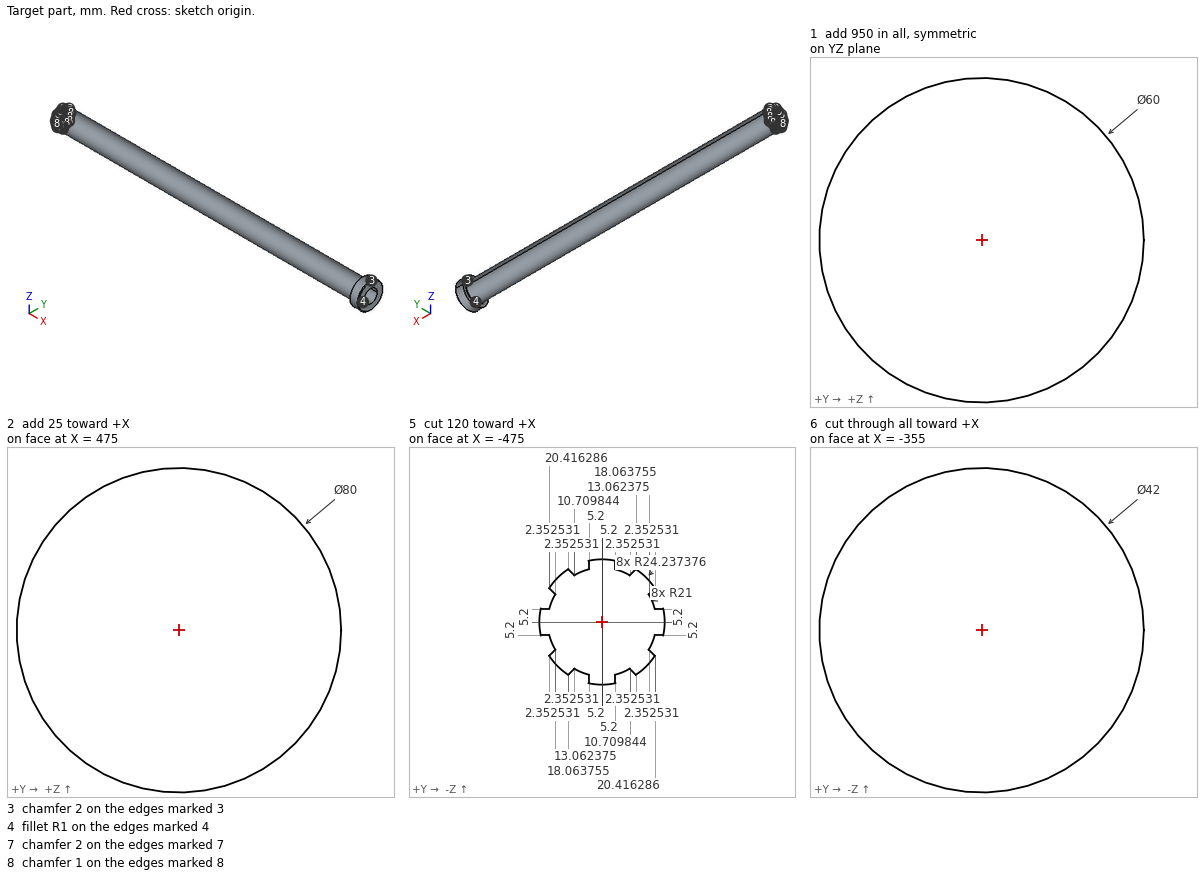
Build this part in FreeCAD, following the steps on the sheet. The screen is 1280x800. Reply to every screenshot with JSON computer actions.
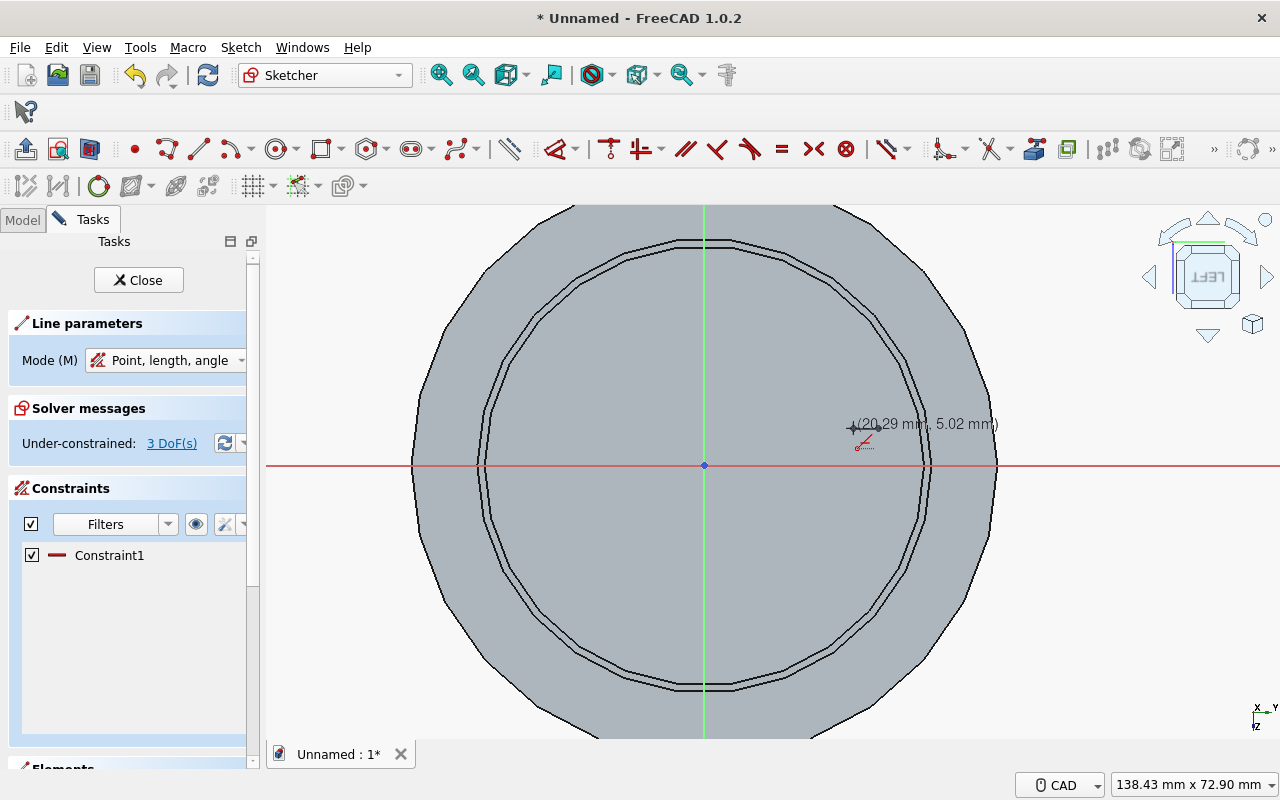
{"action": "left_click", "coordinate": [837, 387]}
{"action": "left_click", "coordinate": [854, 370]}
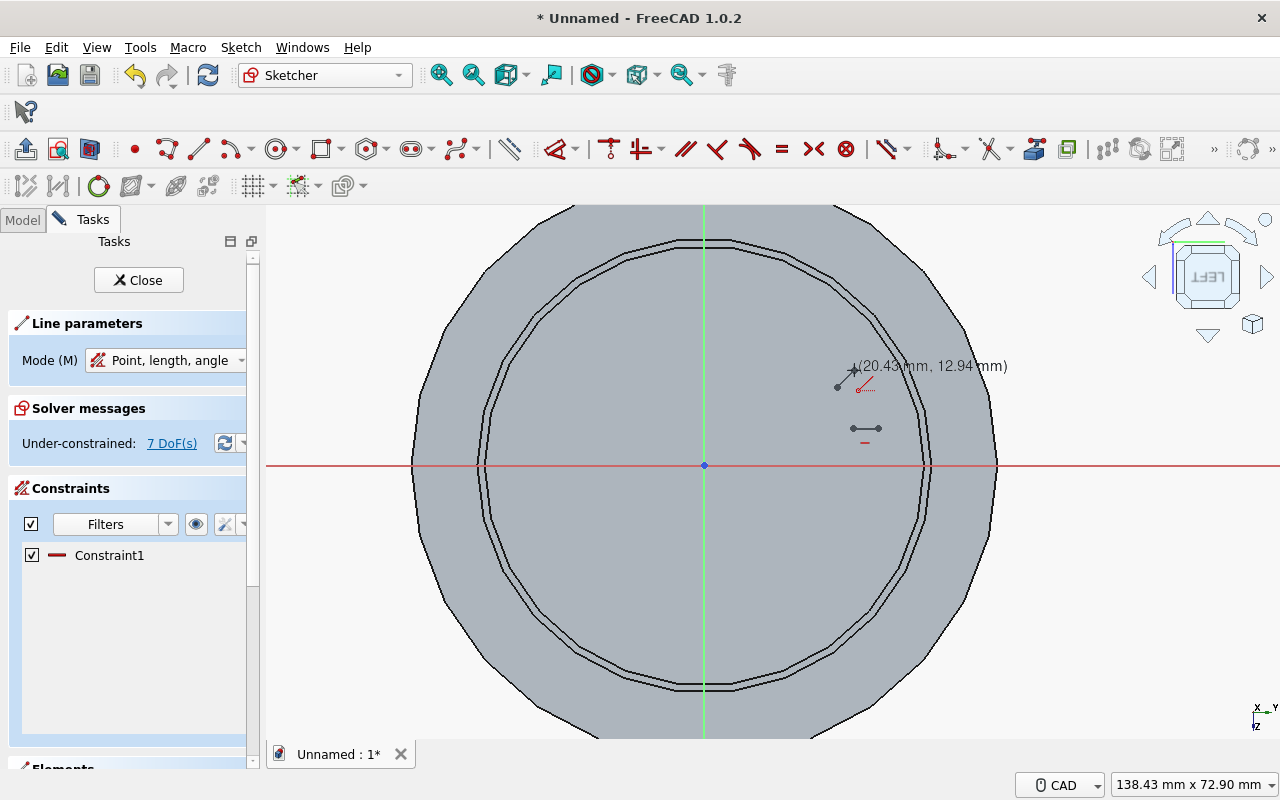
{"action": "left_click", "coordinate": [800, 316]}
{"action": "left_click", "coordinate": [783, 333]}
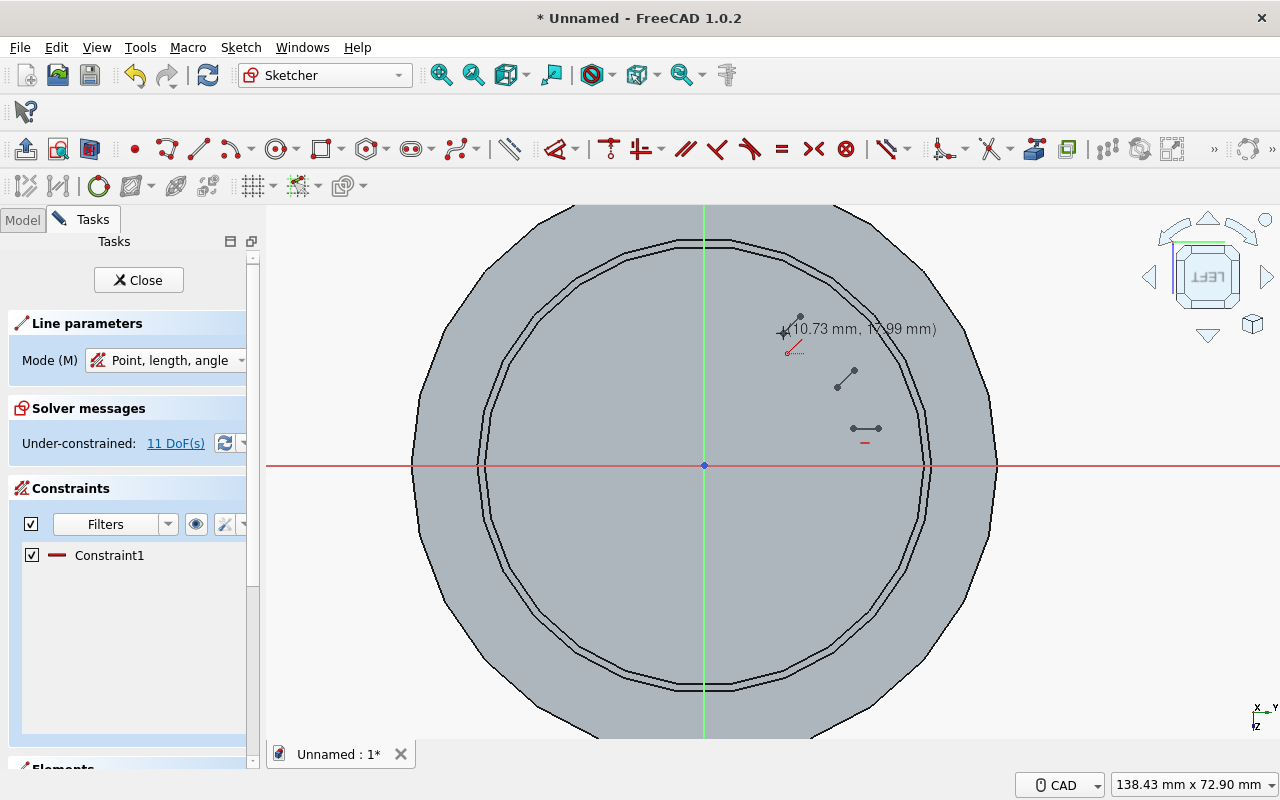
{"action": "left_click", "coordinate": [742, 317]}
{"action": "left_click", "coordinate": [742, 292]}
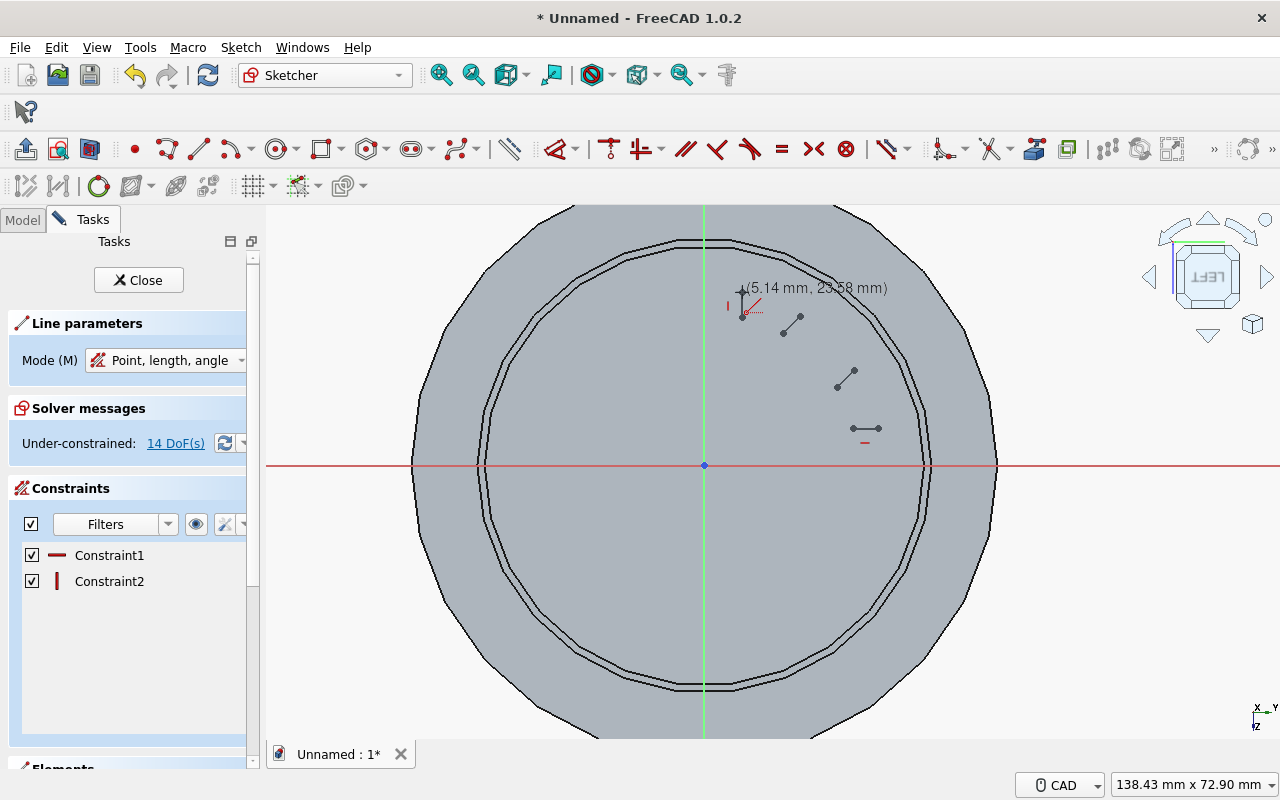
{"action": "left_click", "coordinate": [666, 292]}
{"action": "left_click", "coordinate": [666, 317]}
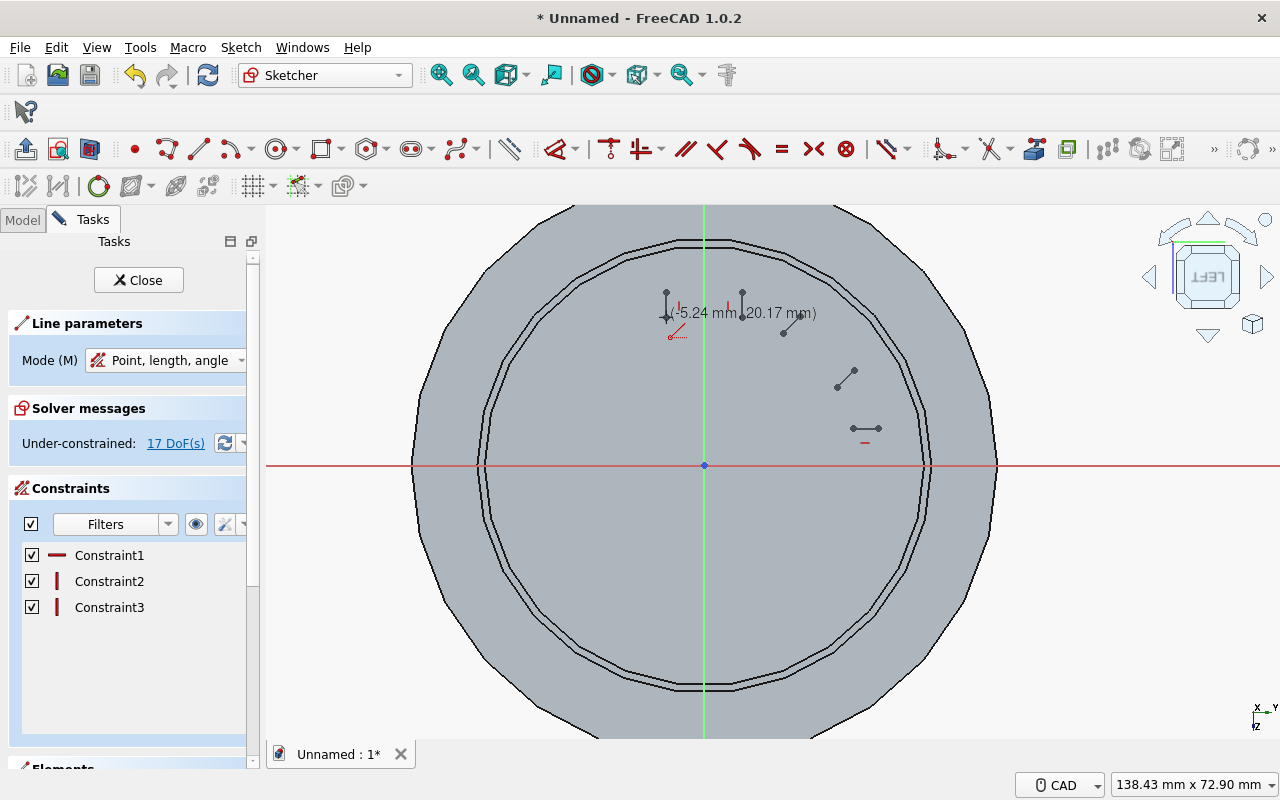
{"action": "left_click", "coordinate": [626, 333]}
{"action": "left_click", "coordinate": [609, 316]}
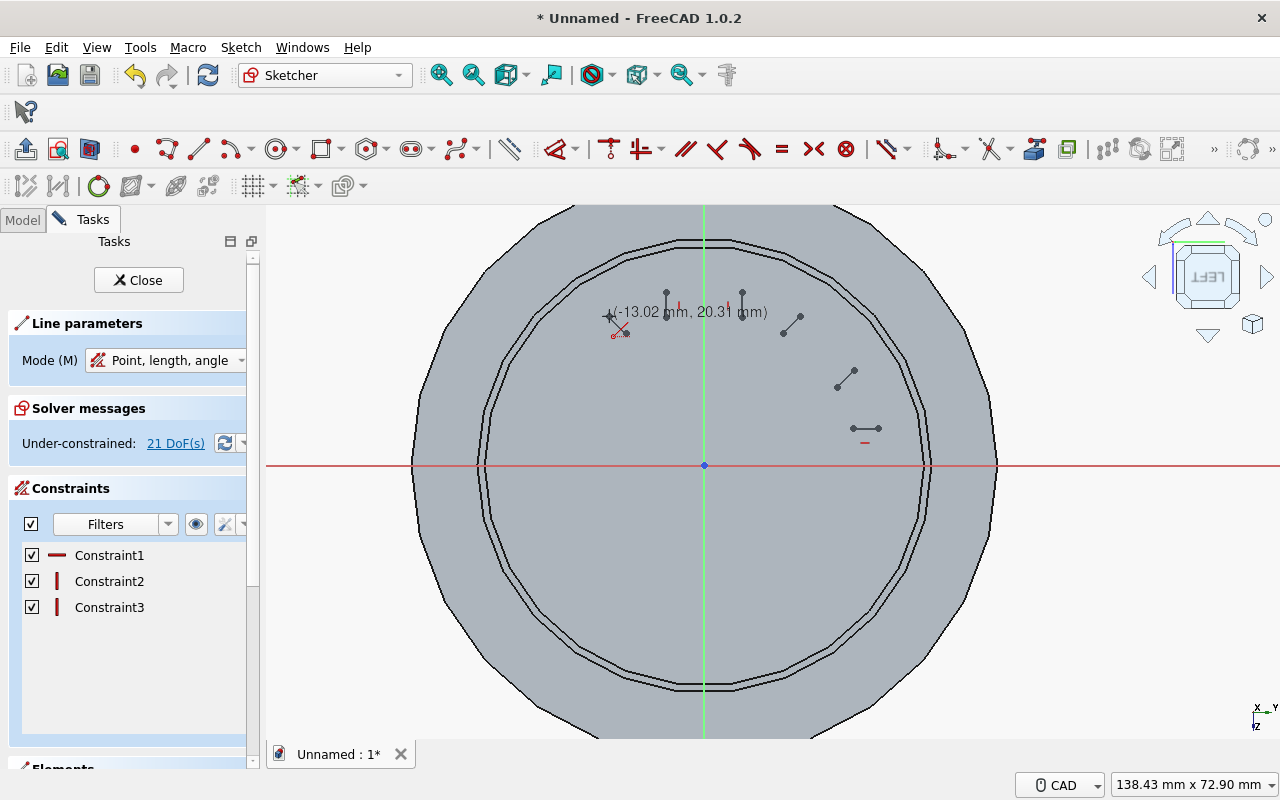
{"action": "left_click", "coordinate": [555, 370]}
{"action": "left_click", "coordinate": [572, 387]}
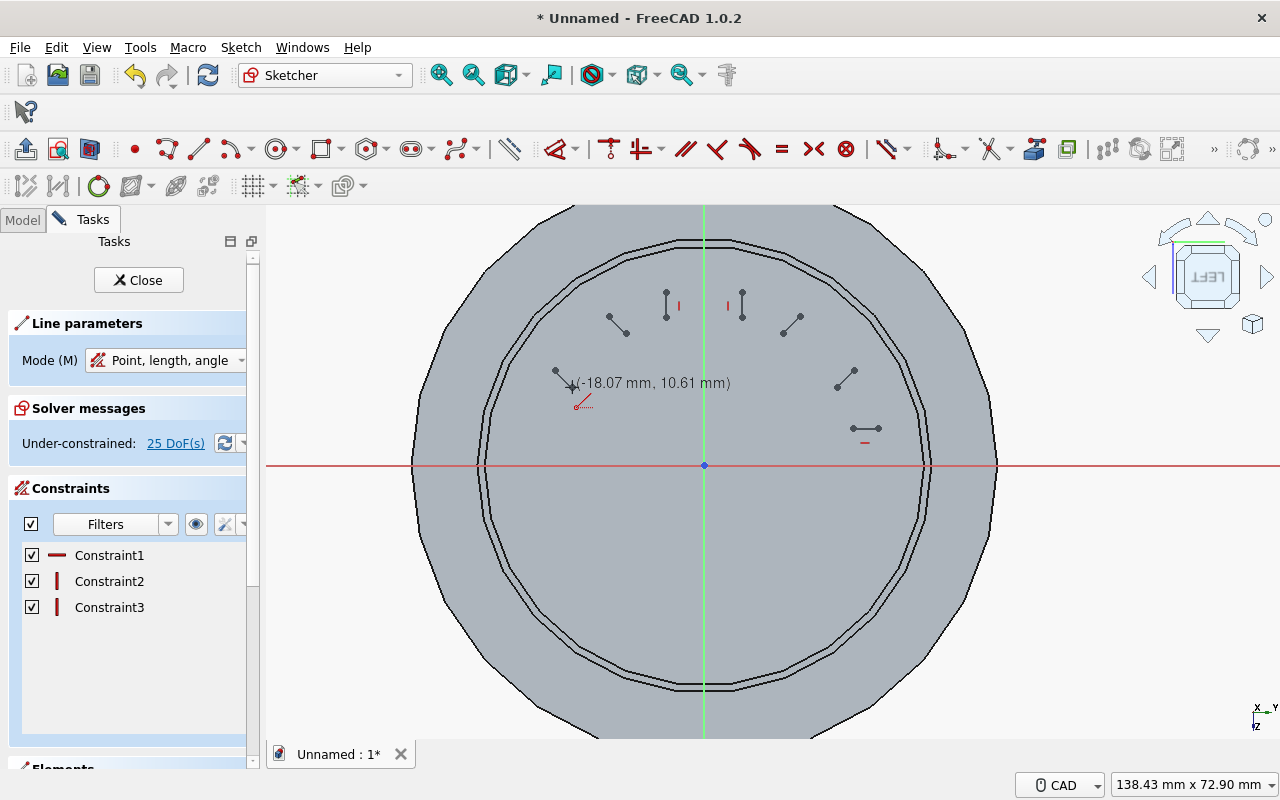
{"action": "left_click", "coordinate": [555, 428]}
{"action": "left_click", "coordinate": [531, 428]}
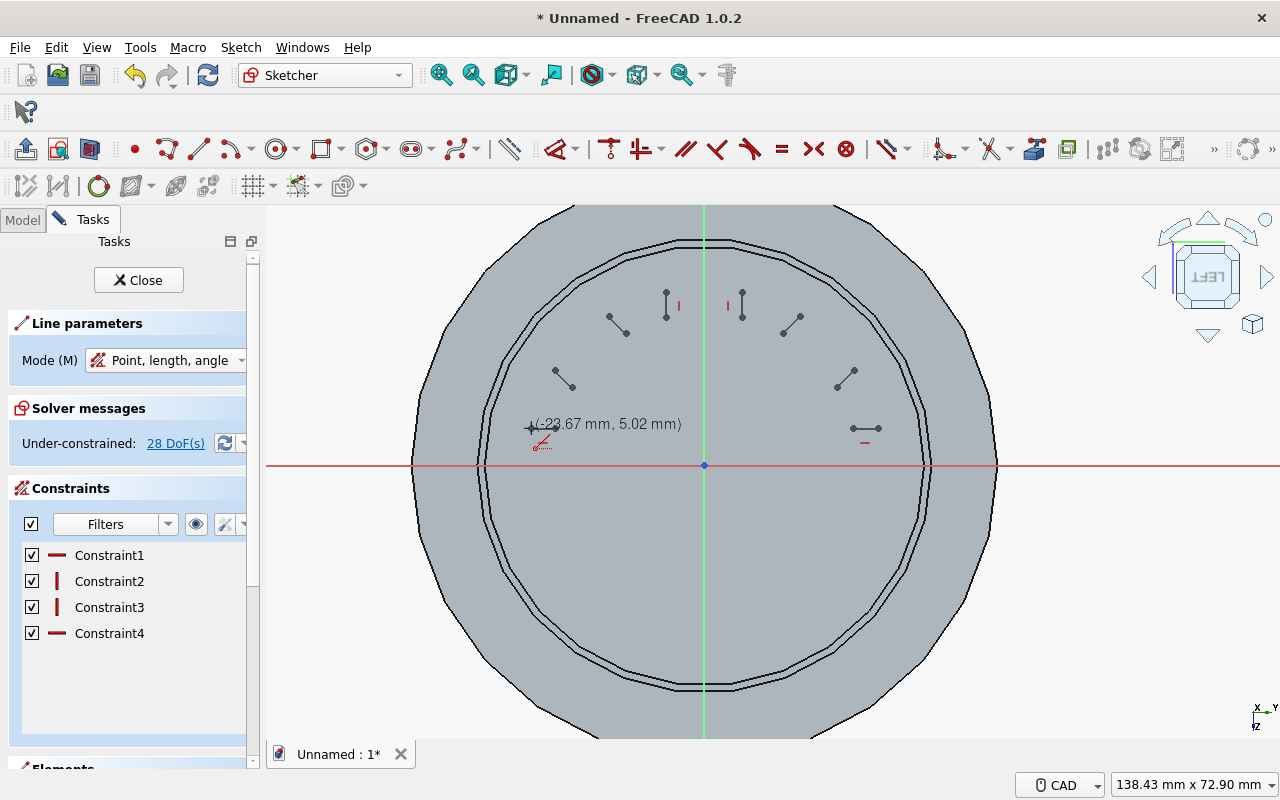
{"action": "left_click", "coordinate": [531, 504]}
{"action": "left_click", "coordinate": [555, 504]}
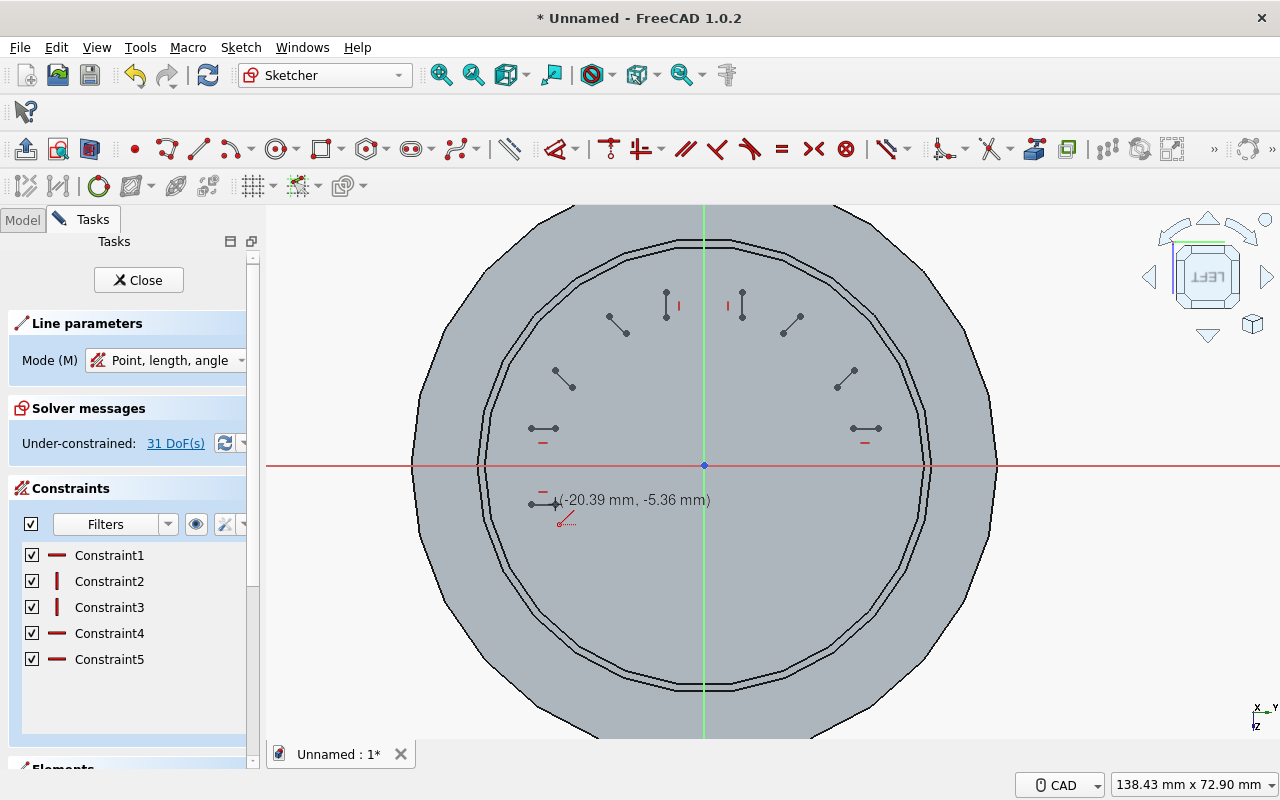
{"action": "left_click", "coordinate": [572, 544]}
{"action": "left_click", "coordinate": [555, 561]}